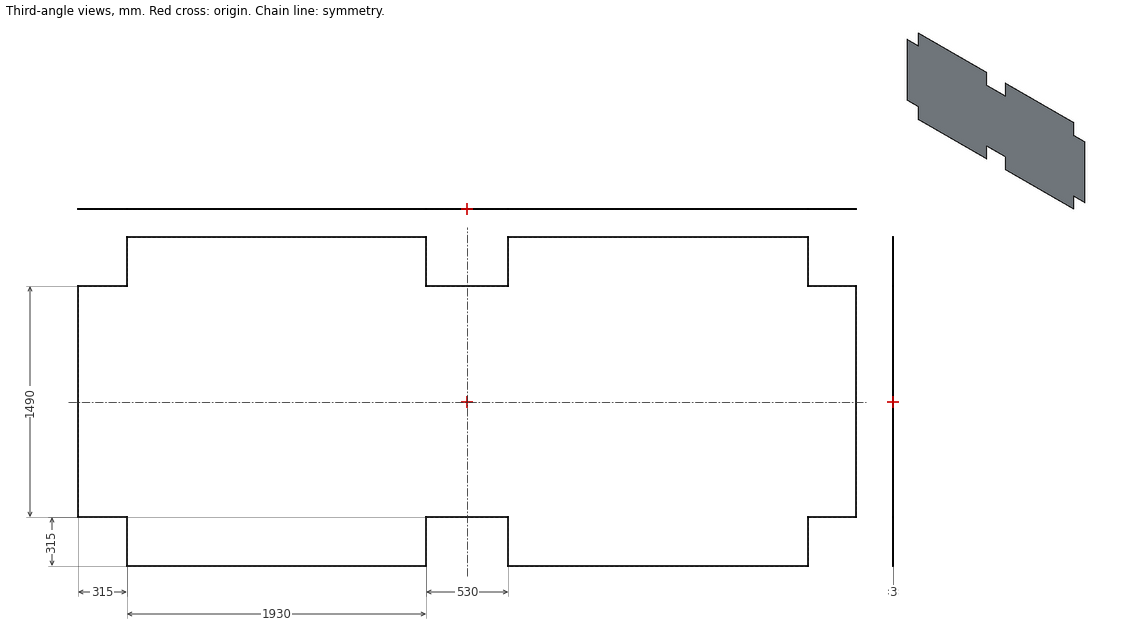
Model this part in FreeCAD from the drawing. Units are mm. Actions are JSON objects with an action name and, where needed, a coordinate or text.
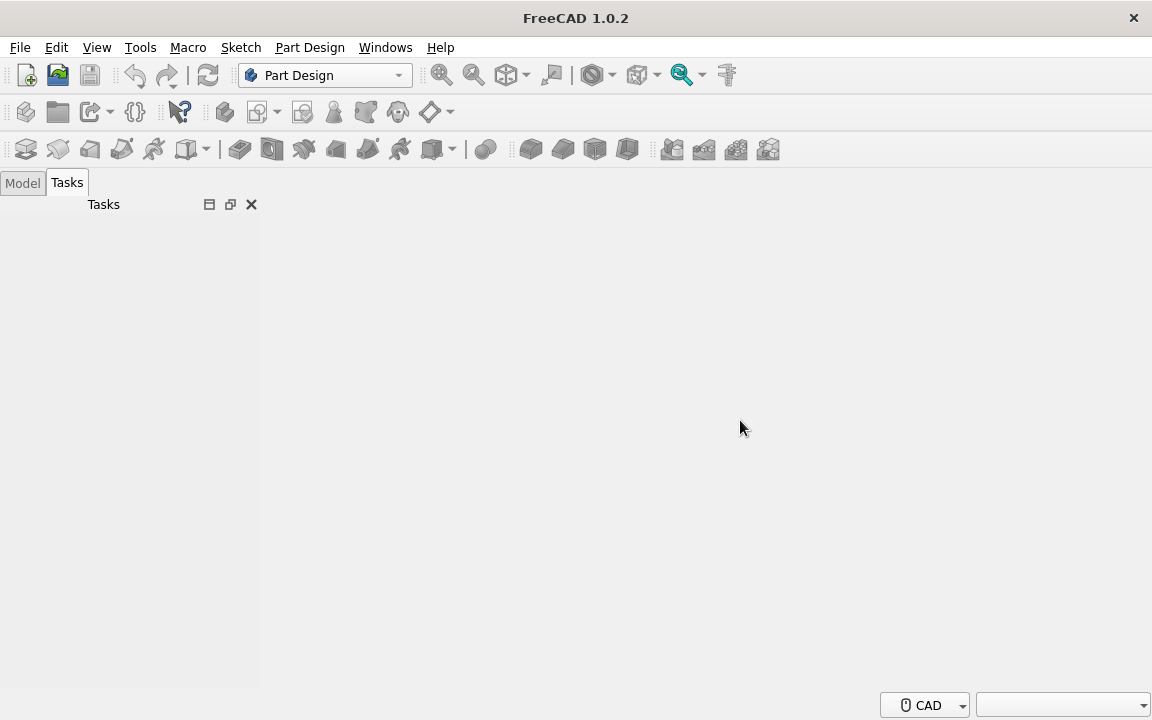
{"action": "left_click", "coordinate": [26, 76]}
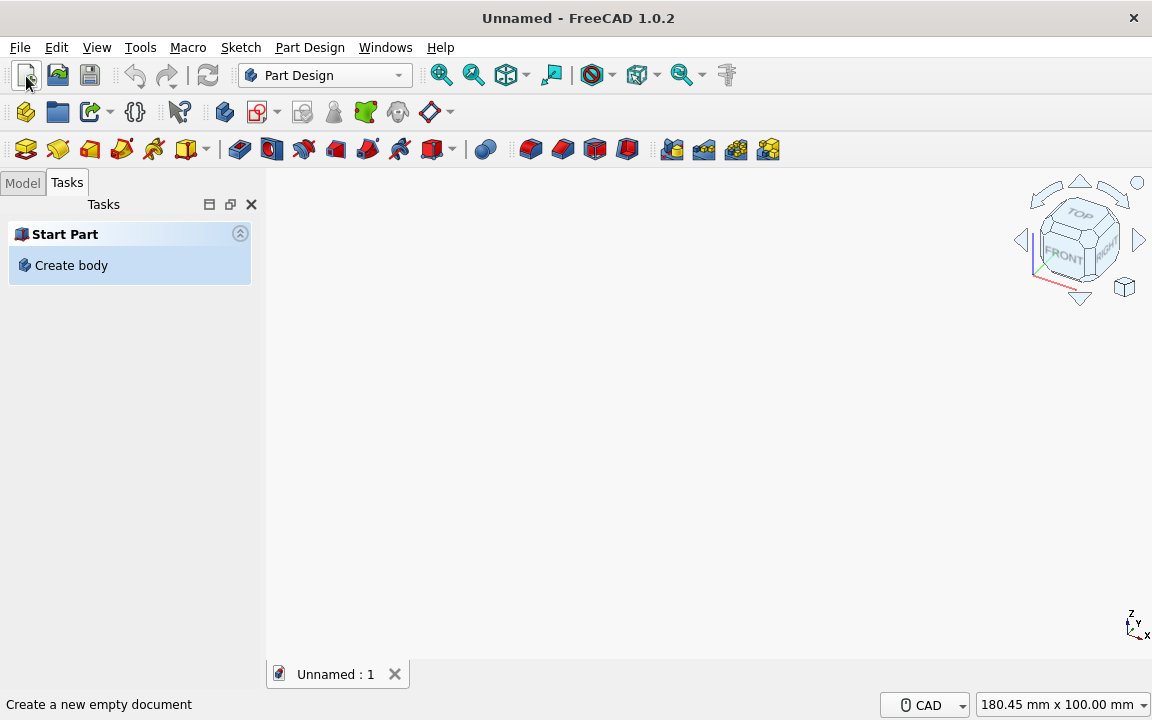
{"action": "left_click", "coordinate": [258, 112]}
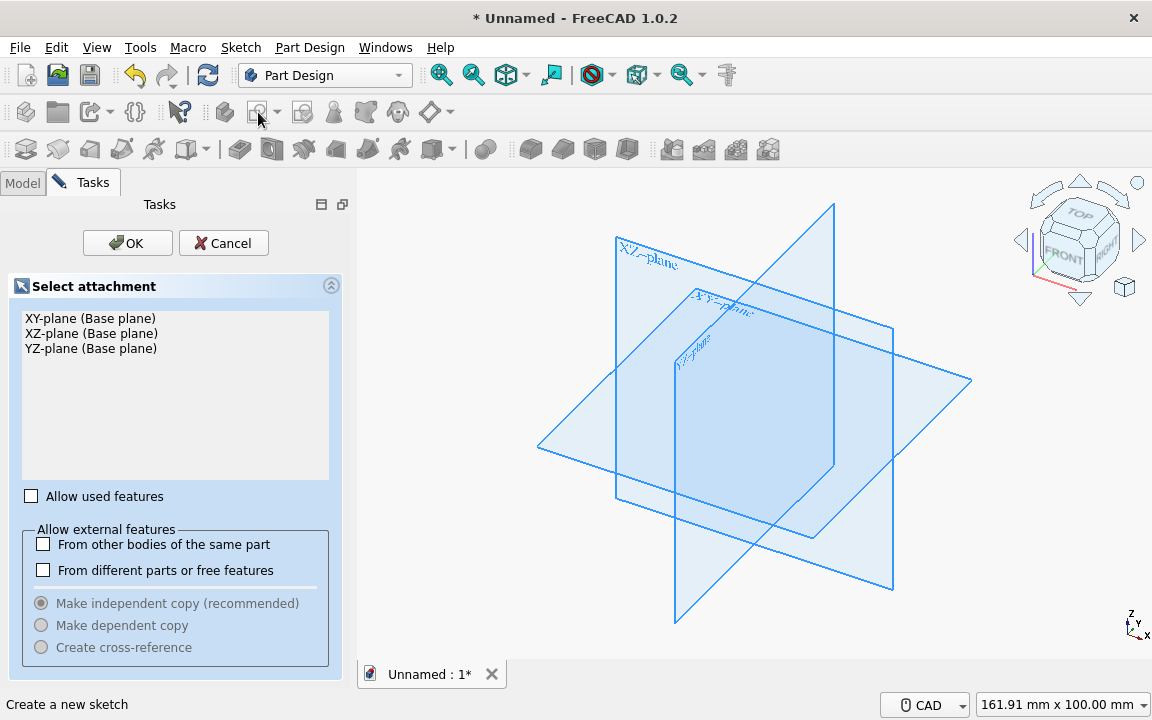
{"action": "left_click", "coordinate": [82, 334]}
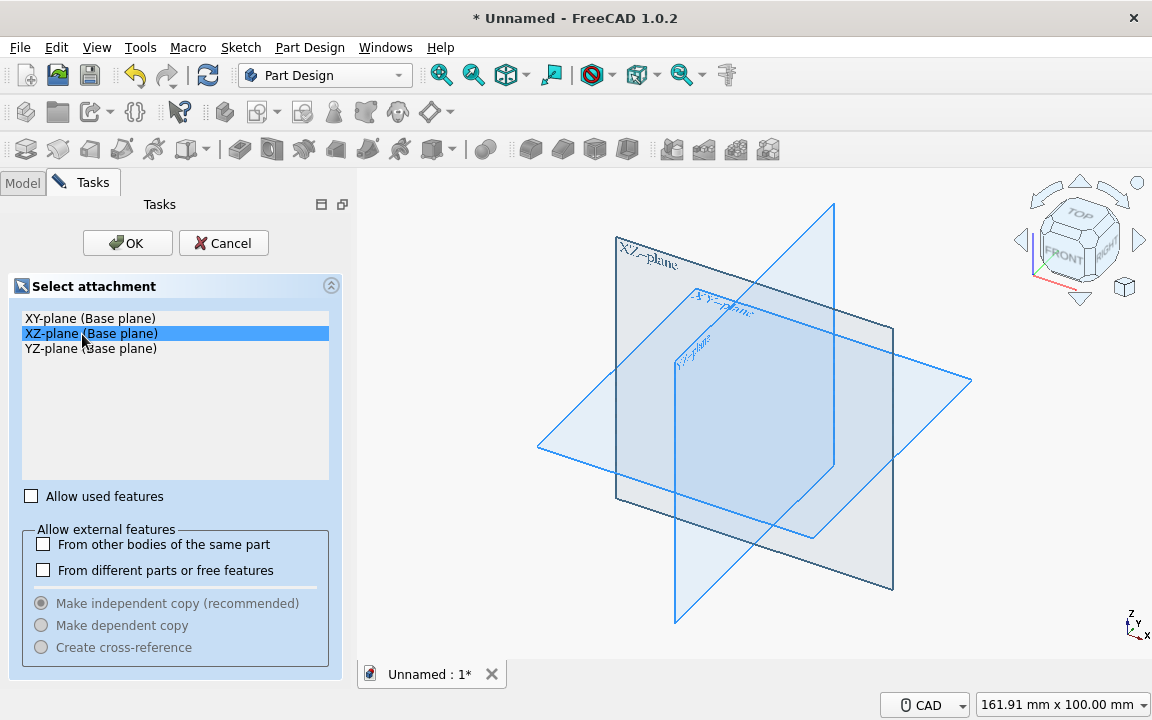
{"action": "left_click", "coordinate": [128, 243]}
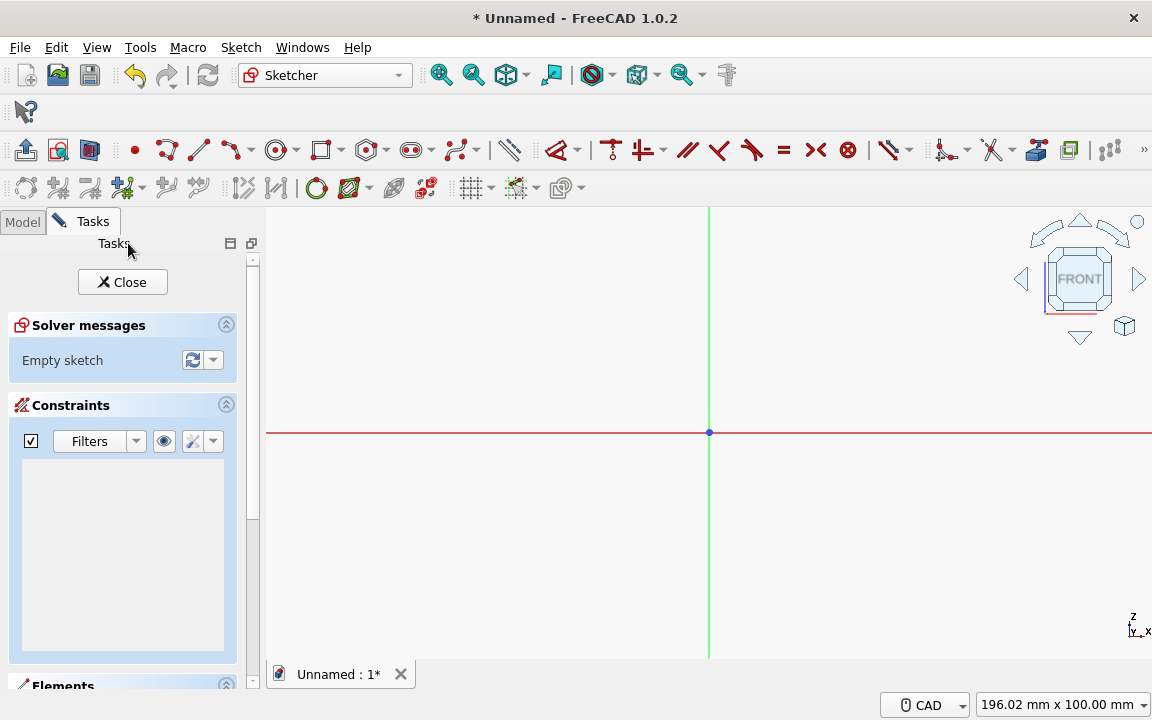
{"action": "scroll", "coordinate": [639, 433], "scroll_direction": "down", "scroll_amount": 18}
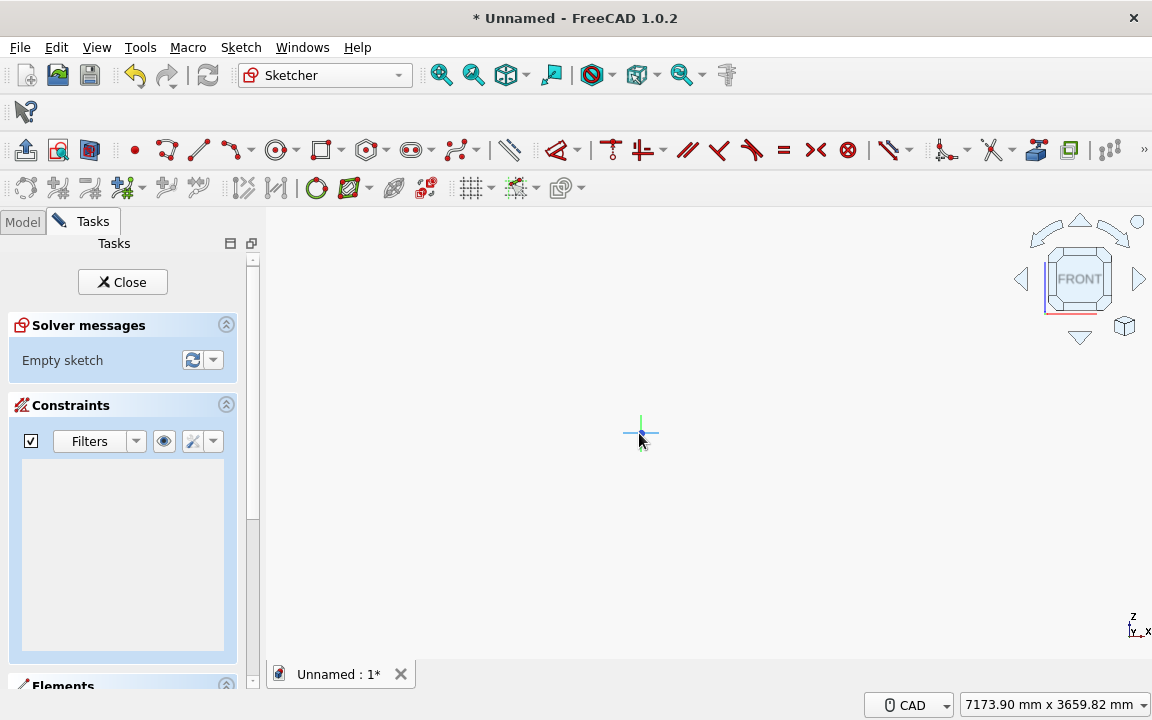
{"action": "left_click", "coordinate": [168, 150]}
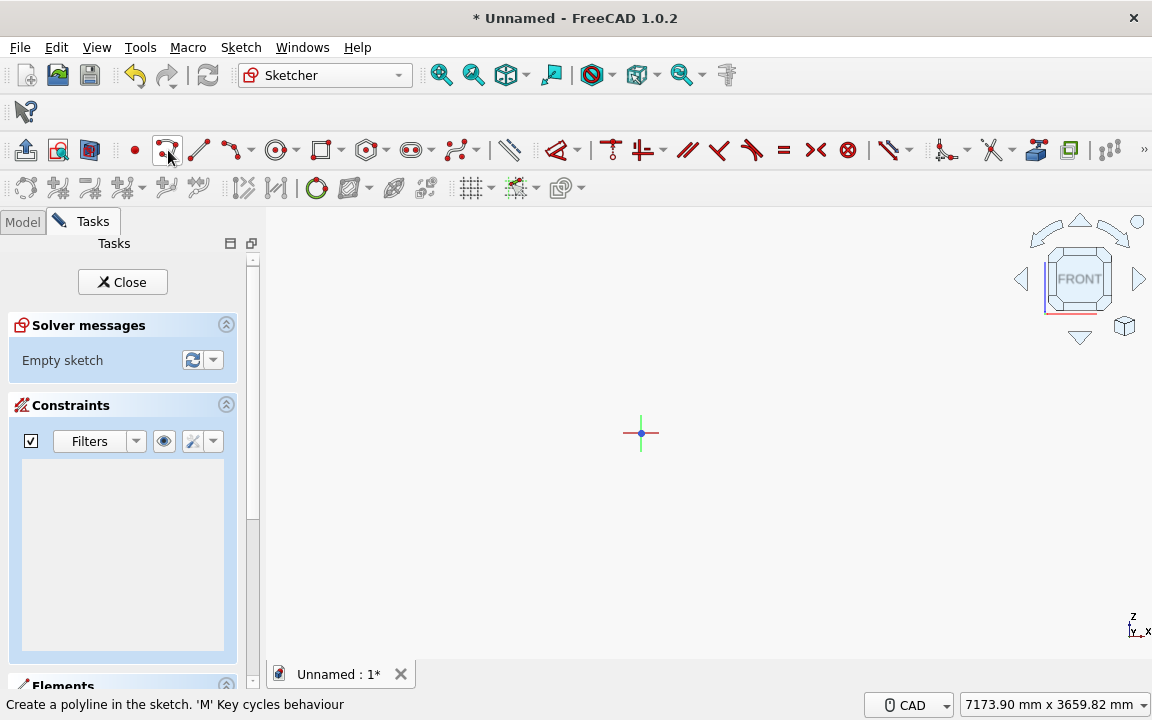
{"action": "left_click", "coordinate": [674, 525]}
{"action": "left_click", "coordinate": [609, 525]}
{"action": "left_click", "coordinate": [609, 564]}
{"action": "left_click", "coordinate": [370, 564]}
{"action": "left_click", "coordinate": [370, 525]}
{"action": "left_click", "coordinate": [331, 525]}
{"action": "left_click", "coordinate": [331, 341]}
{"action": "left_click", "coordinate": [370, 341]}
{"action": "left_click", "coordinate": [370, 303]}
{"action": "left_click", "coordinate": [609, 303]}
{"action": "left_click", "coordinate": [609, 341]}
{"action": "left_click", "coordinate": [674, 341]}
{"action": "left_click", "coordinate": [674, 303]}
{"action": "left_click", "coordinate": [912, 303]}
{"action": "left_click", "coordinate": [912, 341]}
{"action": "left_click", "coordinate": [951, 341]}
{"action": "left_click", "coordinate": [951, 525]}
{"action": "left_click", "coordinate": [912, 525]}
{"action": "left_click", "coordinate": [912, 564]}
{"action": "left_click", "coordinate": [674, 564]}
{"action": "left_click", "coordinate": [674, 526]}
{"action": "key", "text": "Escape"}
{"action": "key", "text": "Escape"}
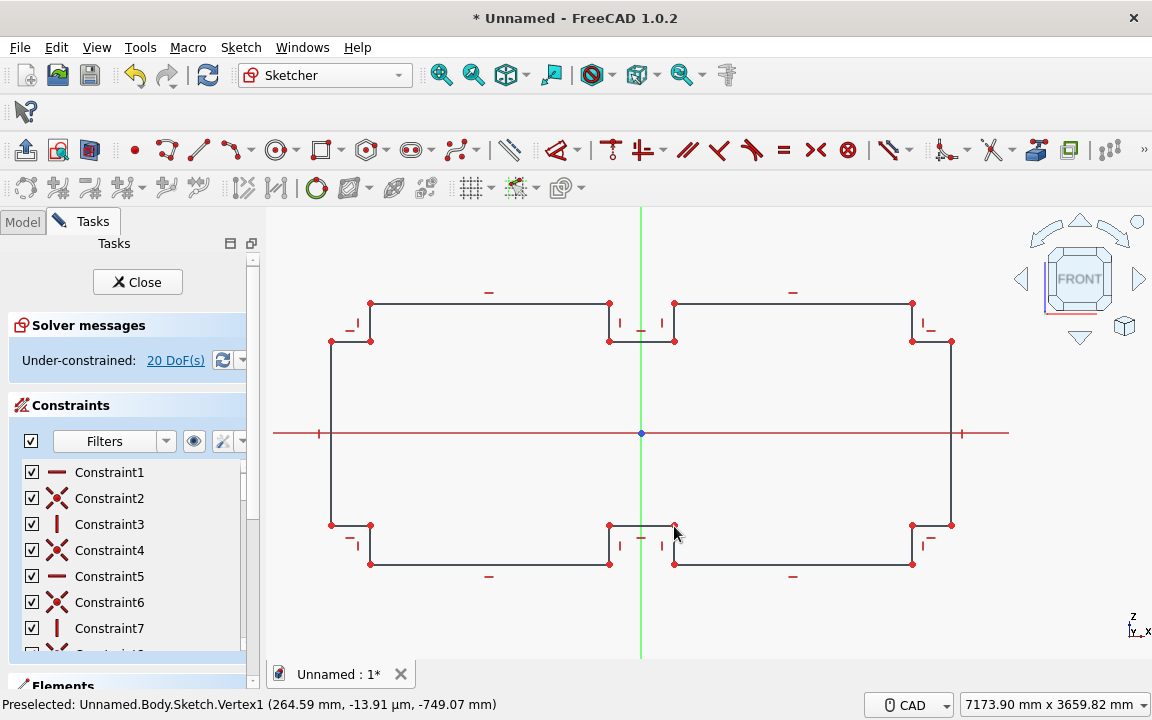
{"action": "left_click", "coordinate": [370, 526]}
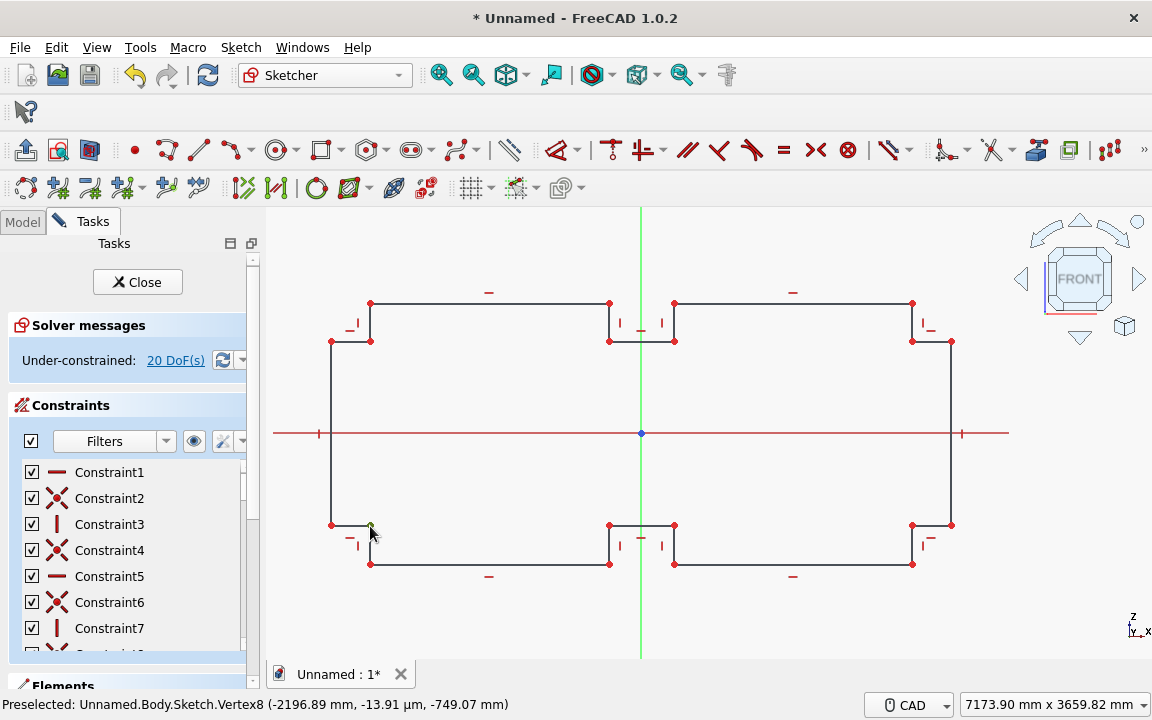
{"action": "left_click", "coordinate": [370, 342]}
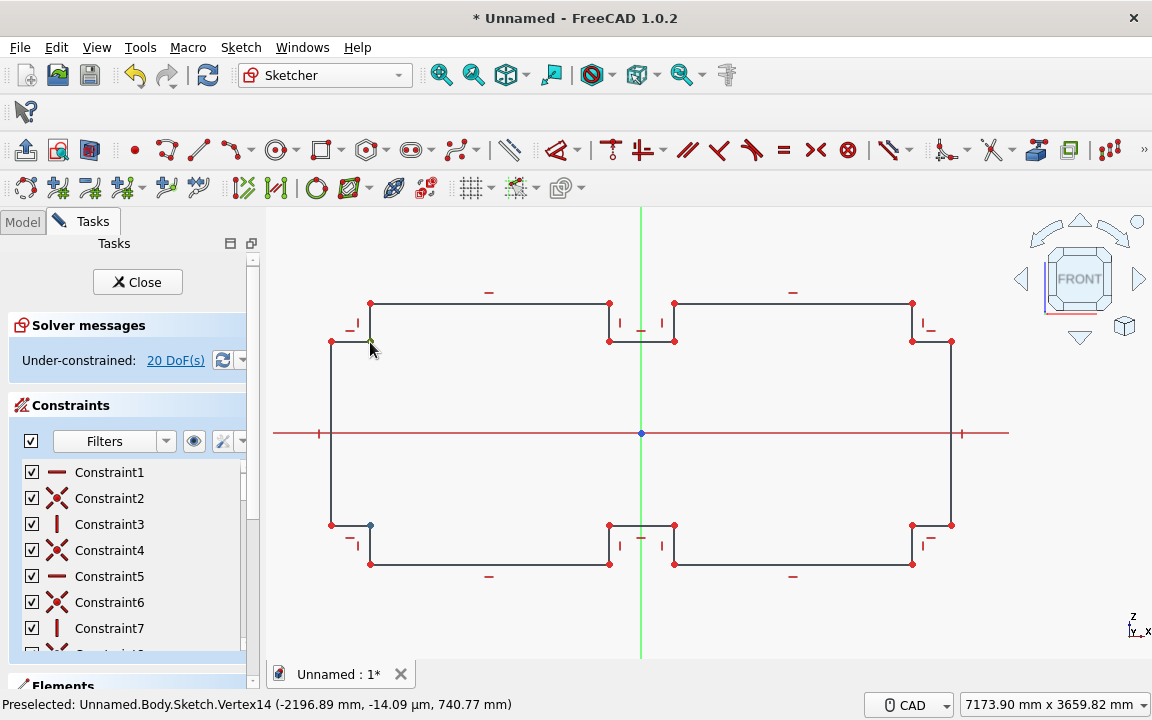
{"action": "left_click", "coordinate": [393, 433]}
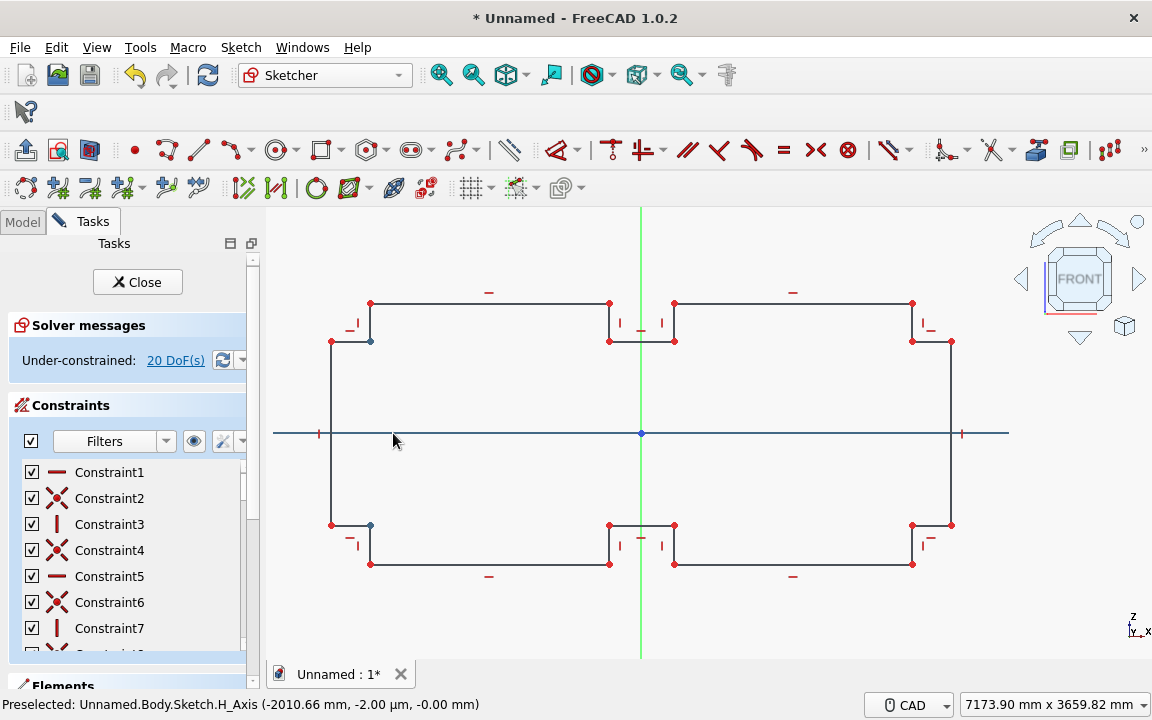
{"action": "key", "text": "s"}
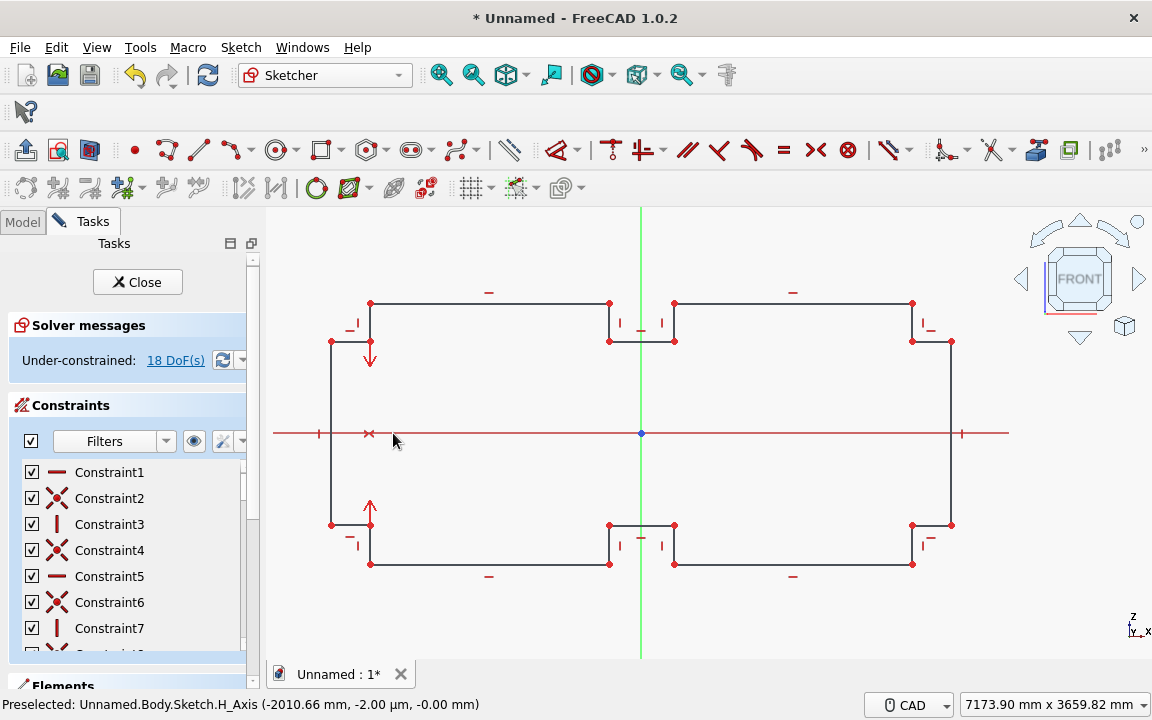
{"action": "left_click", "coordinate": [609, 565]}